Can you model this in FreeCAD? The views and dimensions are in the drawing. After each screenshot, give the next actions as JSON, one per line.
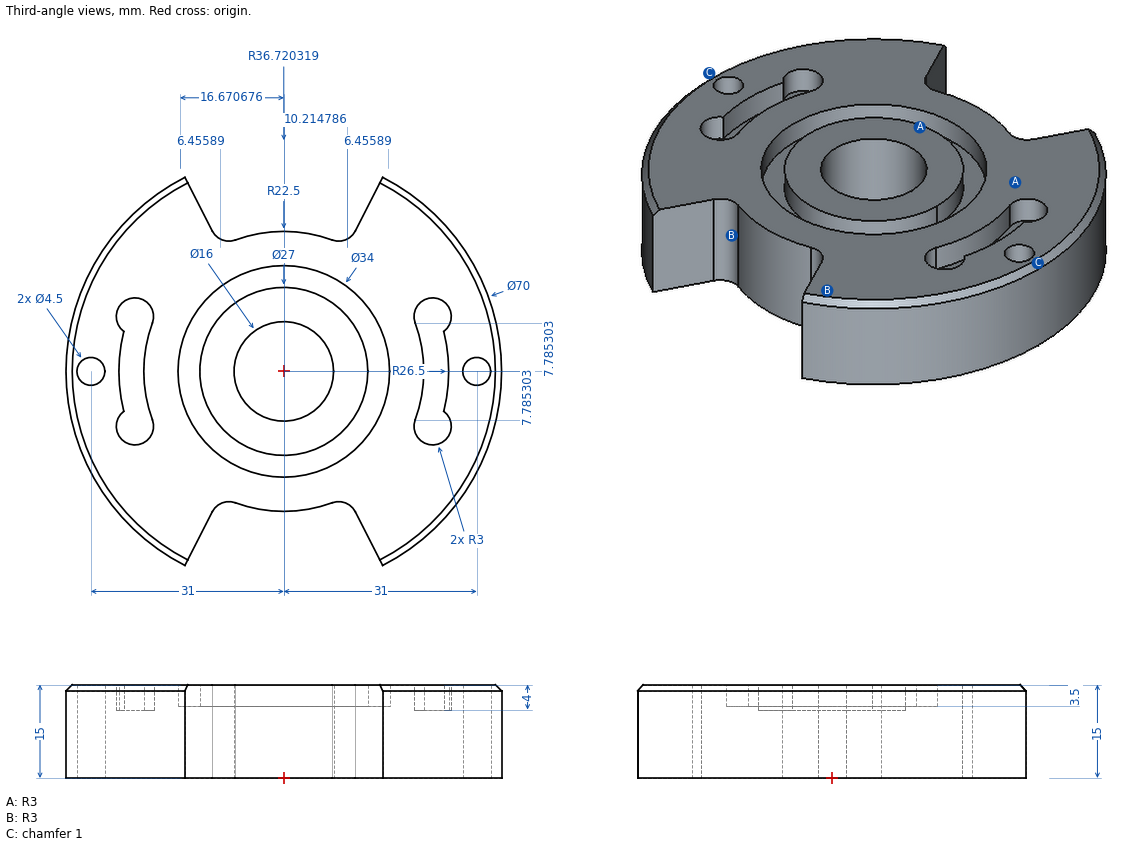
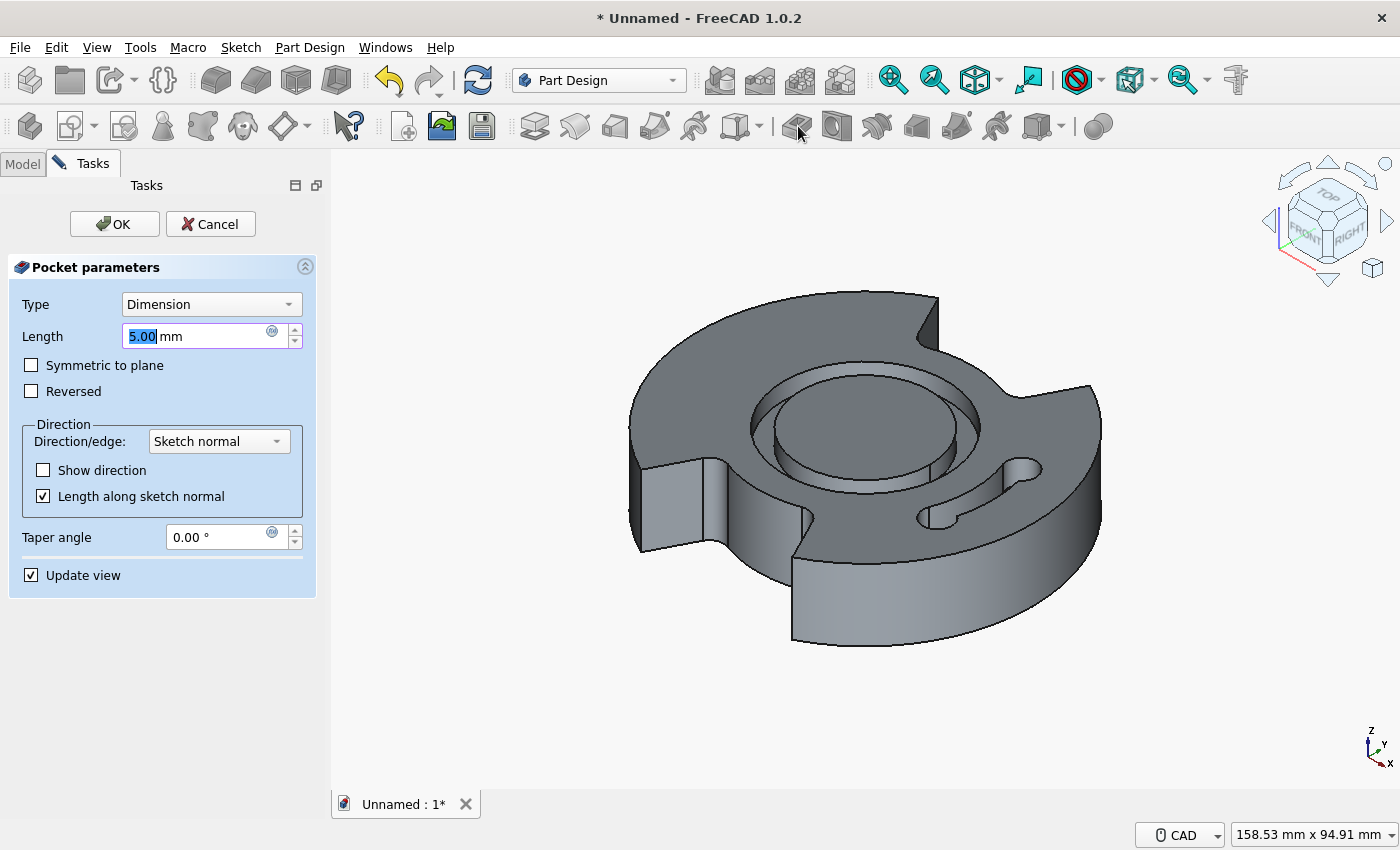
{"action": "type", "text": "4"}
{"action": "key", "text": "Tab"}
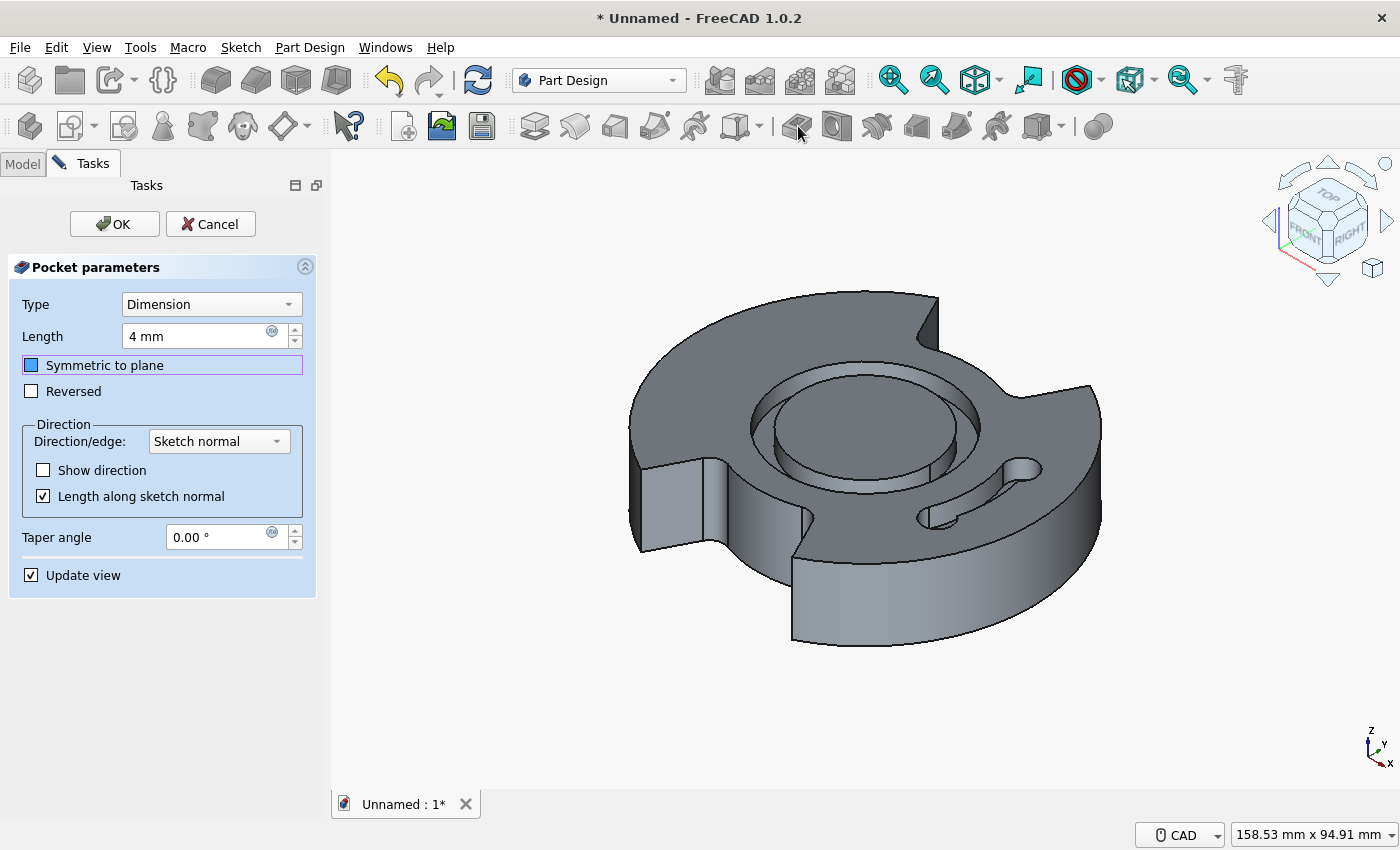
{"action": "left_click", "coordinate": [115, 224]}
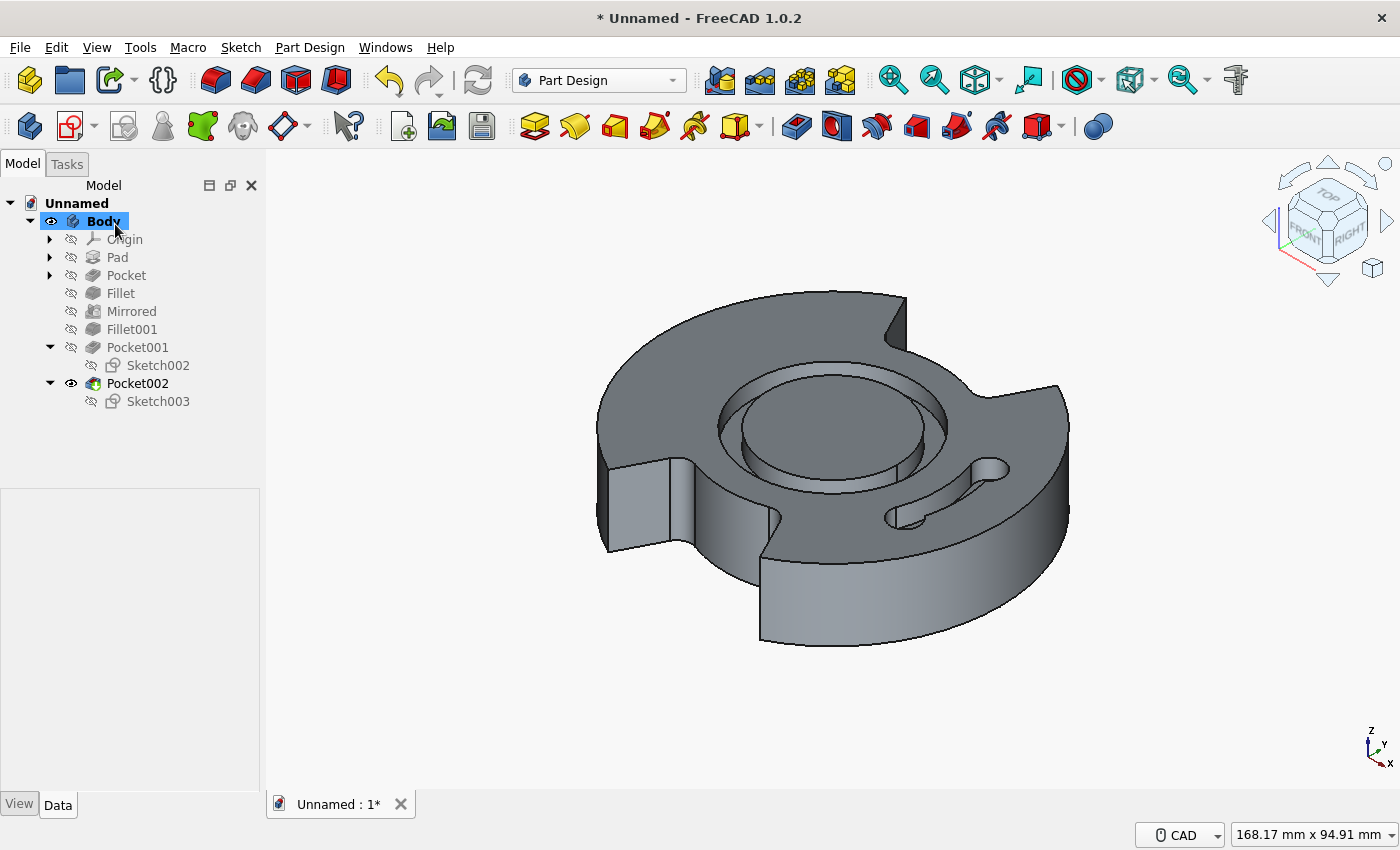
{"action": "left_click", "coordinate": [116, 383]}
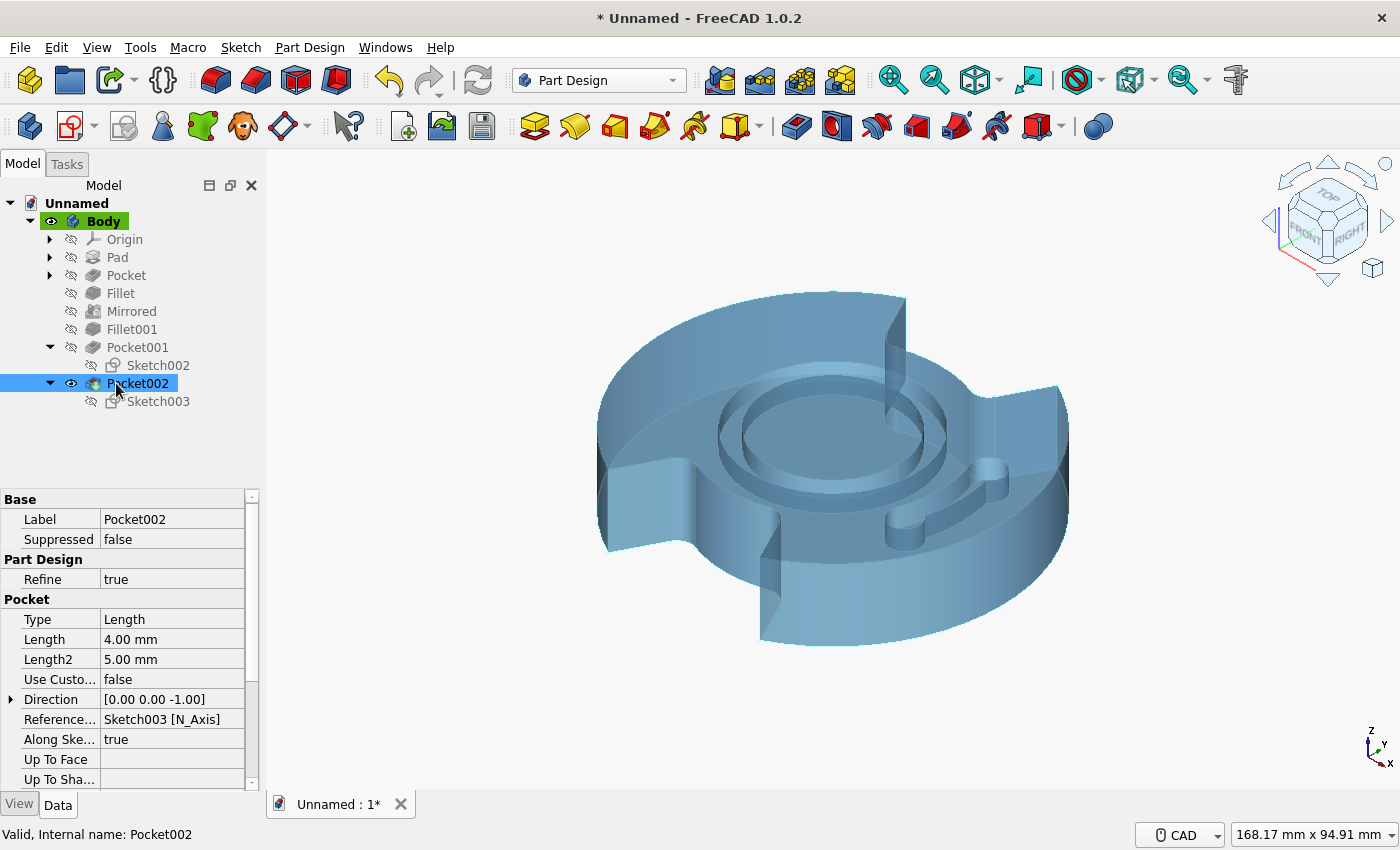
{"action": "left_click", "coordinate": [720, 80]}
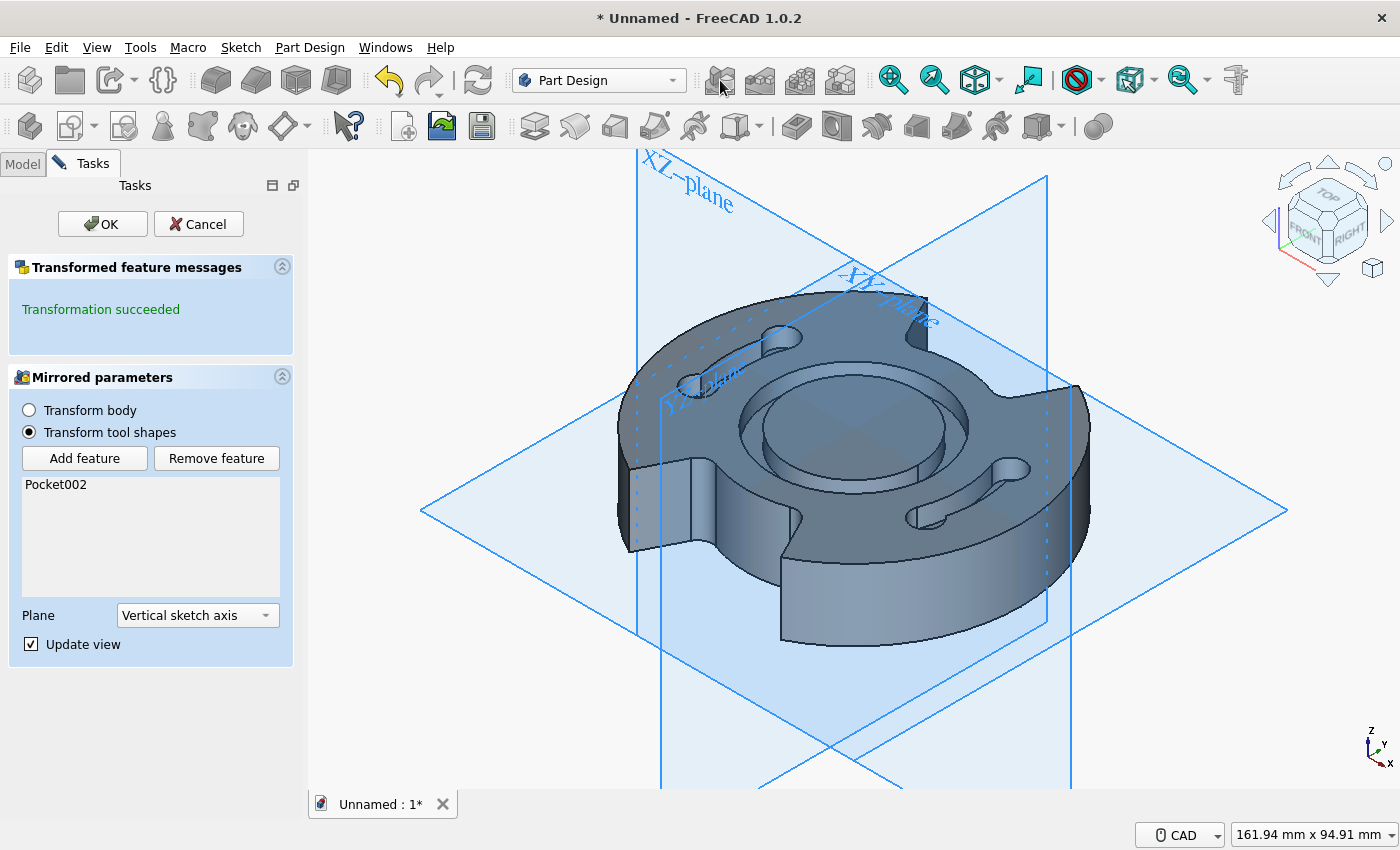
{"action": "left_click", "coordinate": [198, 616]}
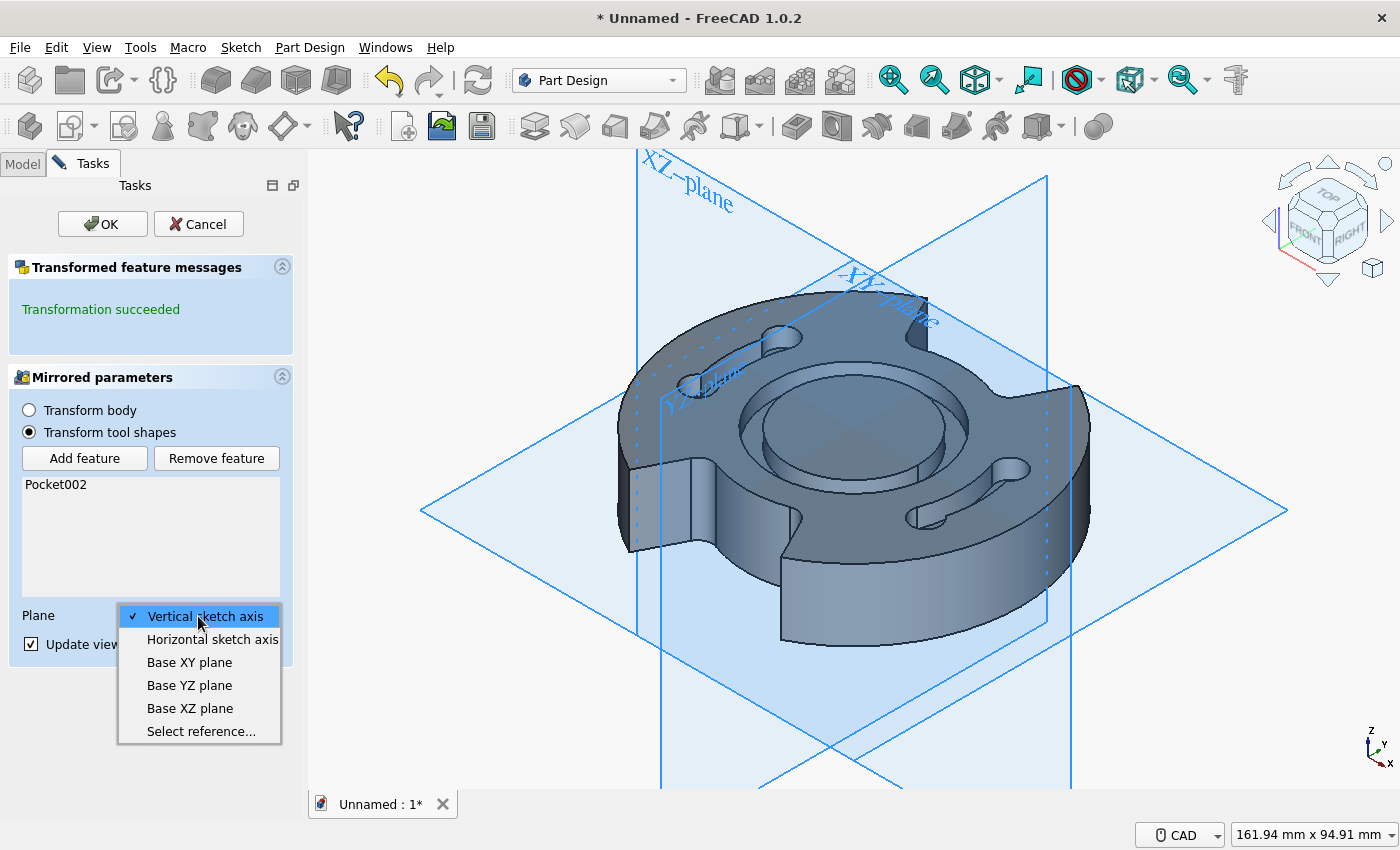
{"action": "left_click", "coordinate": [198, 686]}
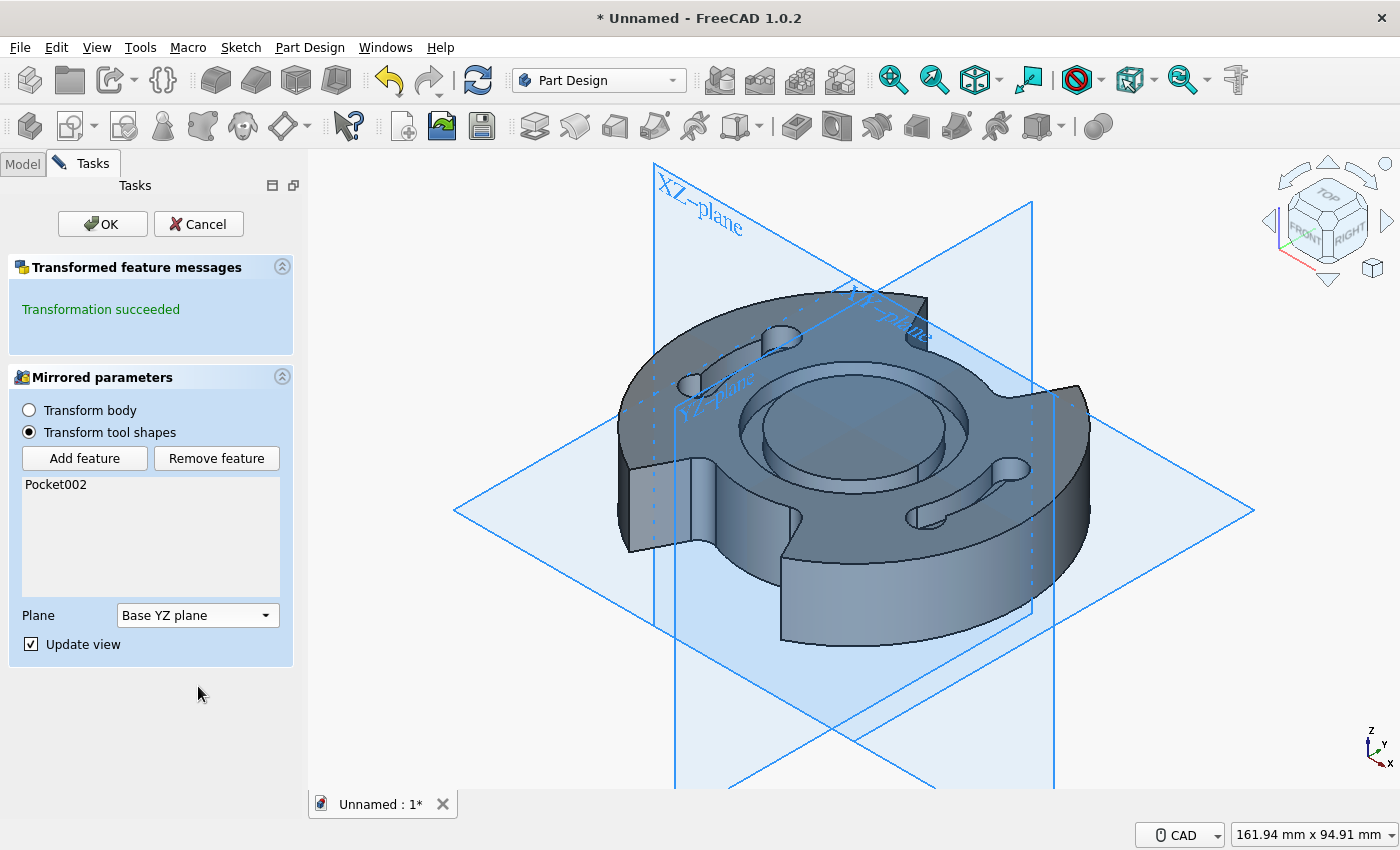
{"action": "left_click", "coordinate": [103, 224]}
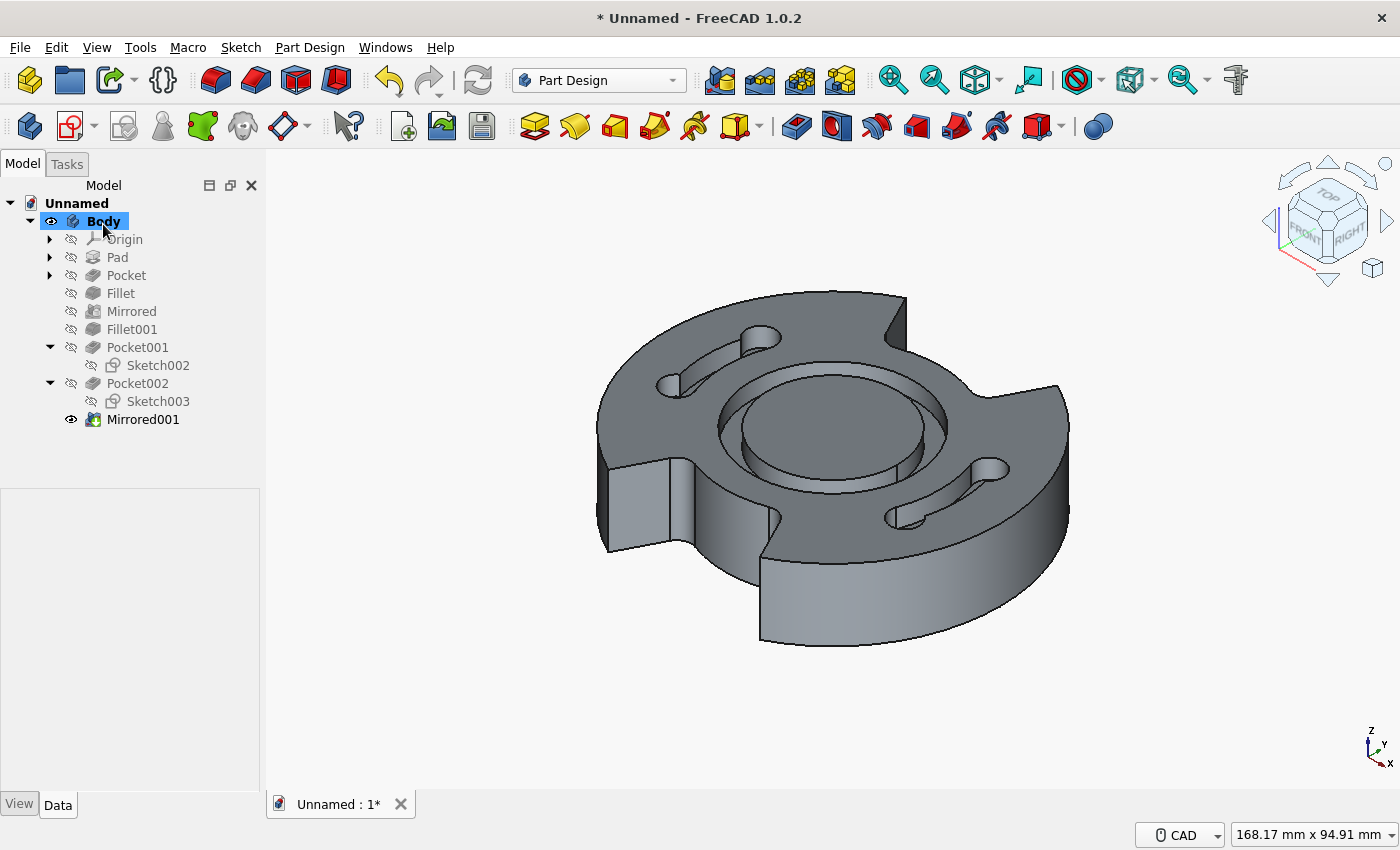
{"action": "left_click", "coordinate": [1013, 433]}